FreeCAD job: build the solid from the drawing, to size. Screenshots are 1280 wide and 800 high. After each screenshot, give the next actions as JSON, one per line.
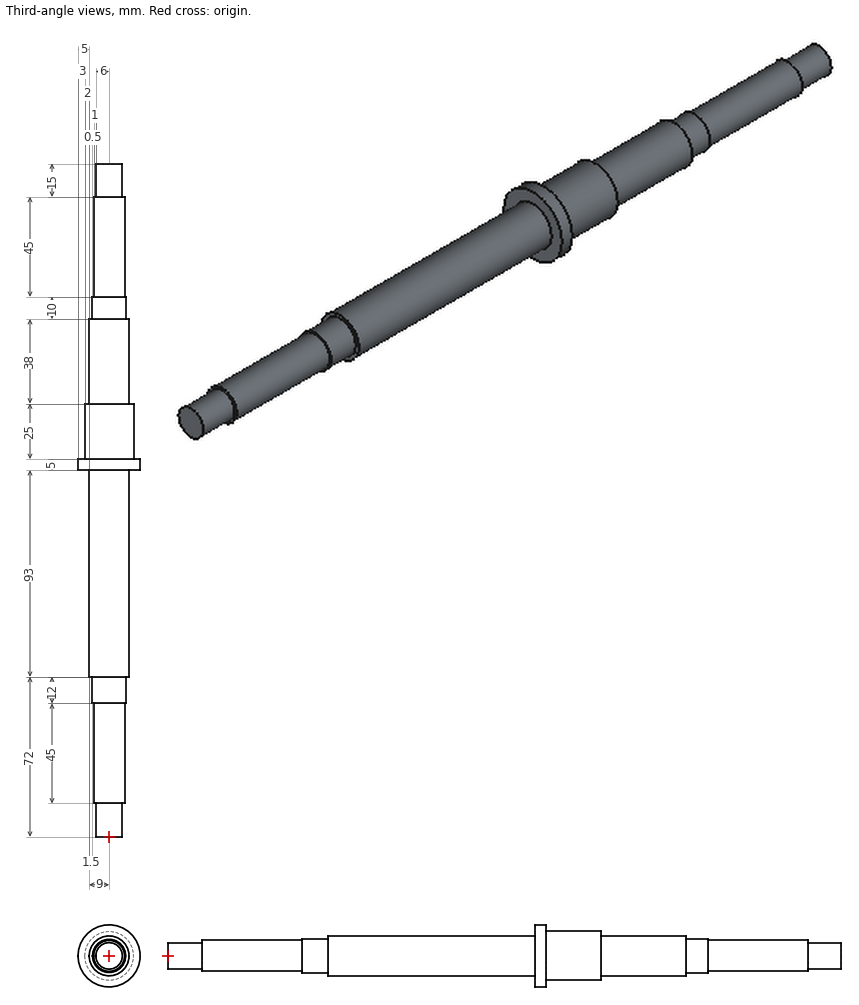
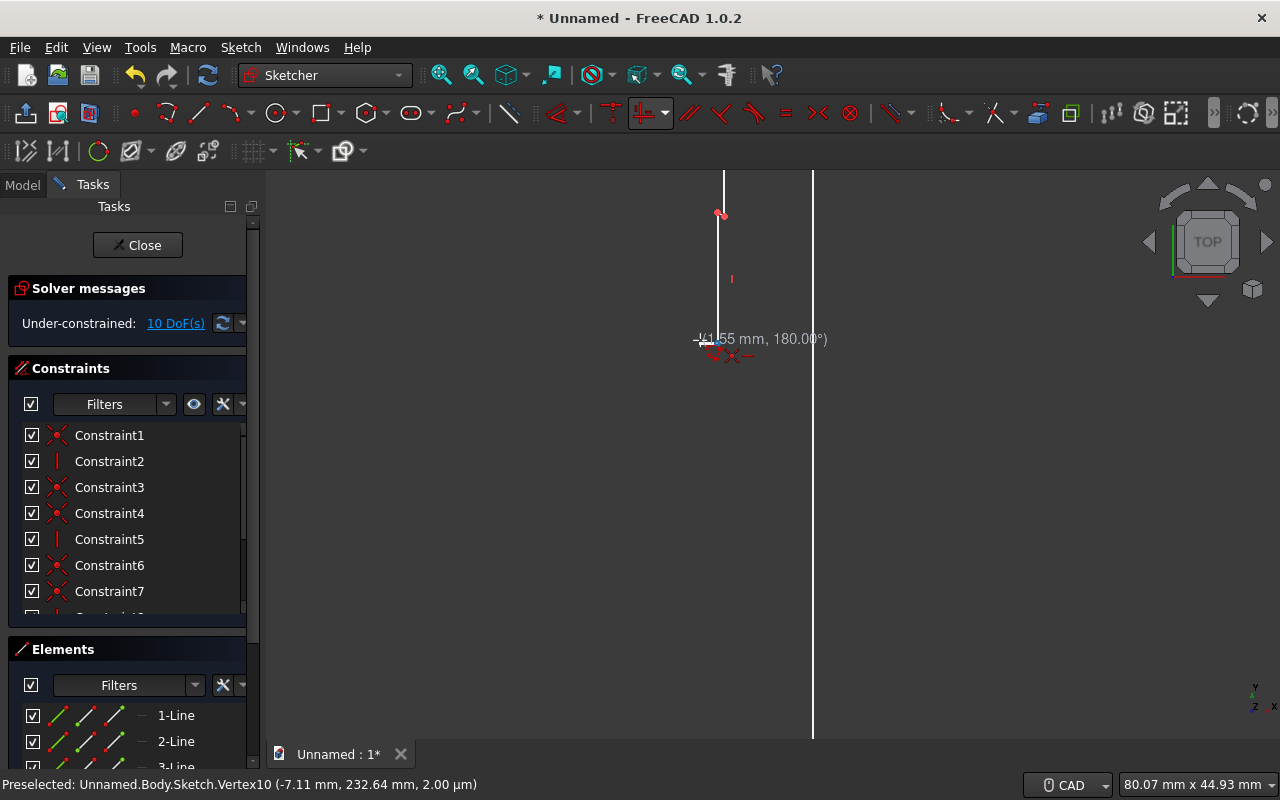
{"action": "left_click", "coordinate": [699, 339]}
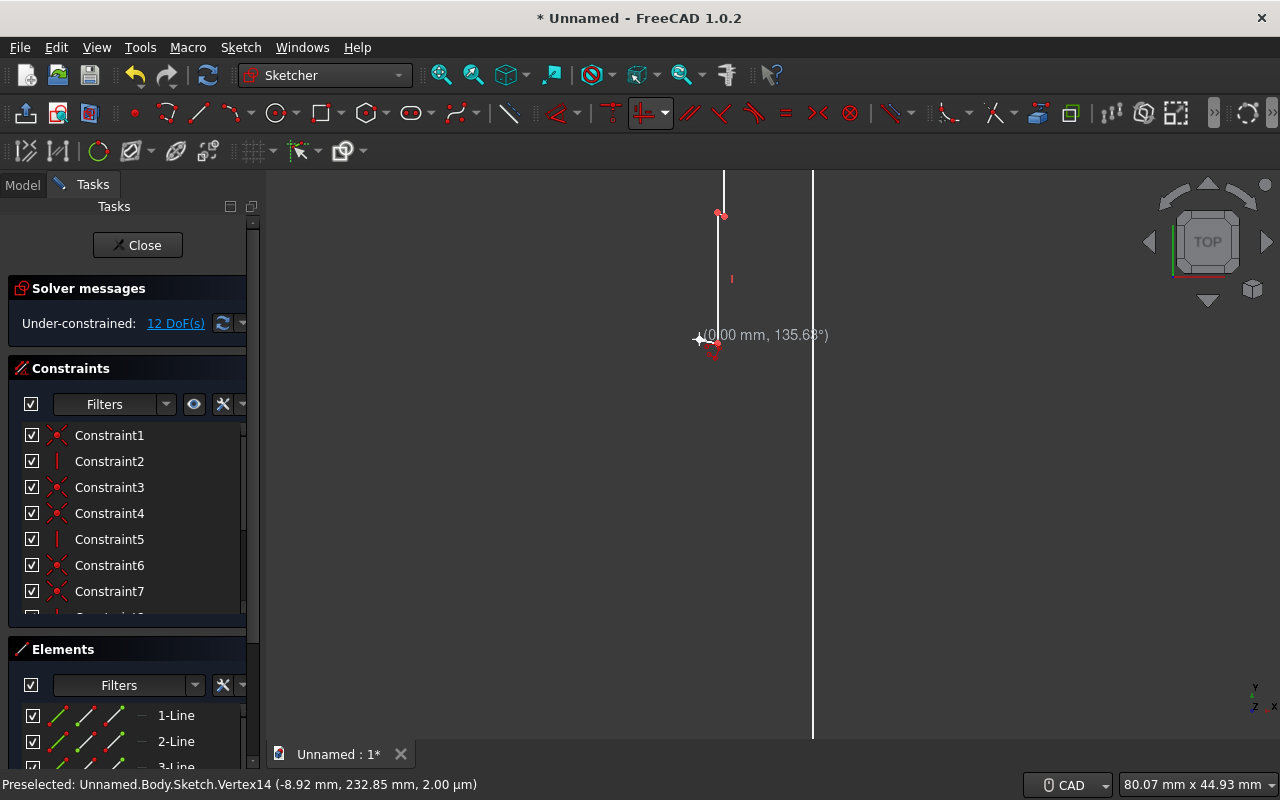
{"action": "scroll", "coordinate": [703, 363], "scroll_direction": "down", "scroll_amount": 12}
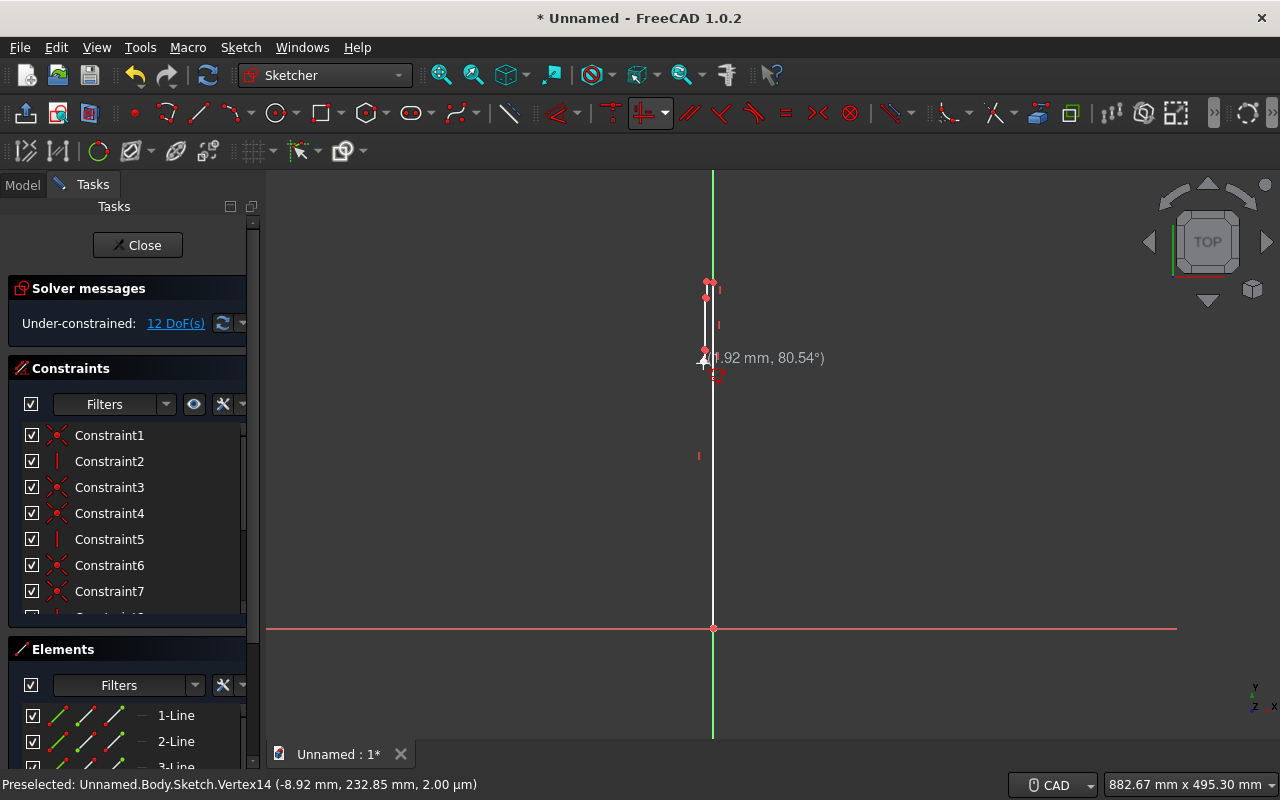
{"action": "scroll", "coordinate": [703, 405], "scroll_direction": "up", "scroll_amount": 3}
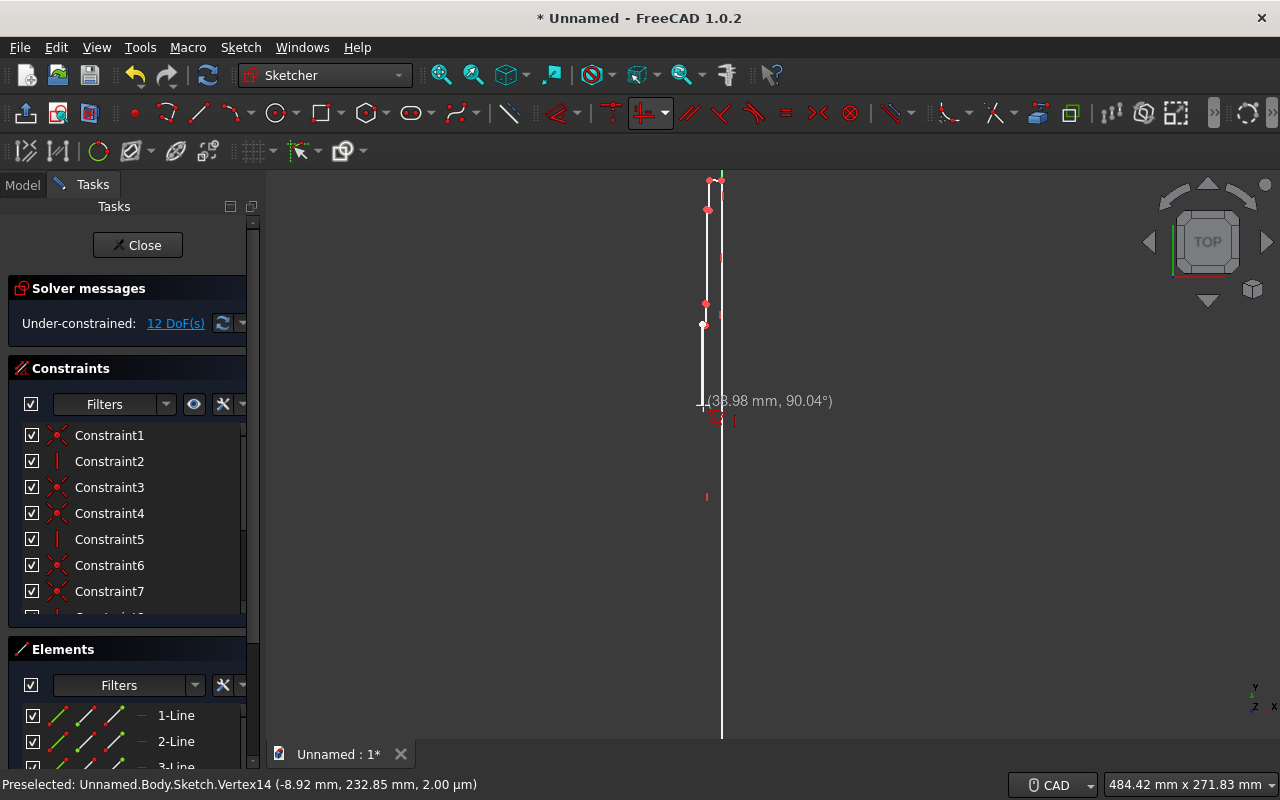
{"action": "left_click", "coordinate": [703, 404]}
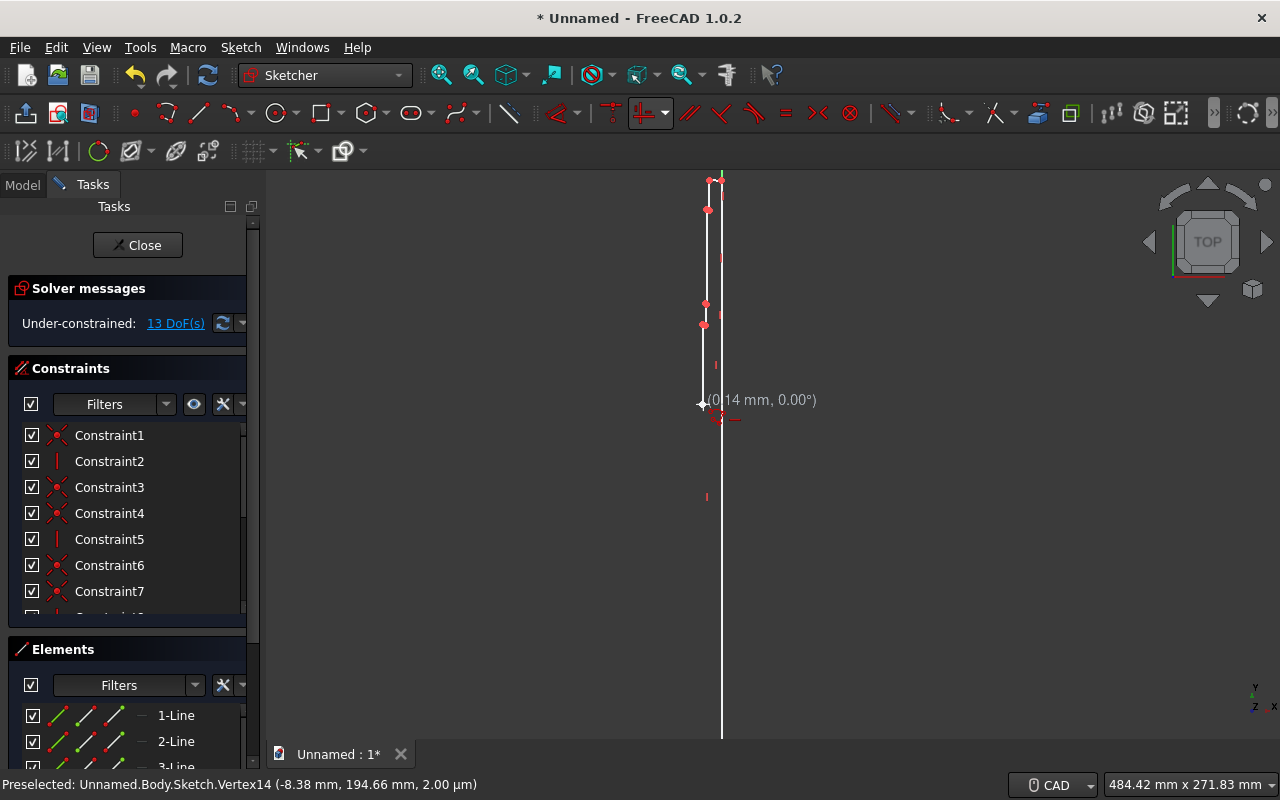
{"action": "scroll", "coordinate": [699, 404], "scroll_direction": "up", "scroll_amount": 7}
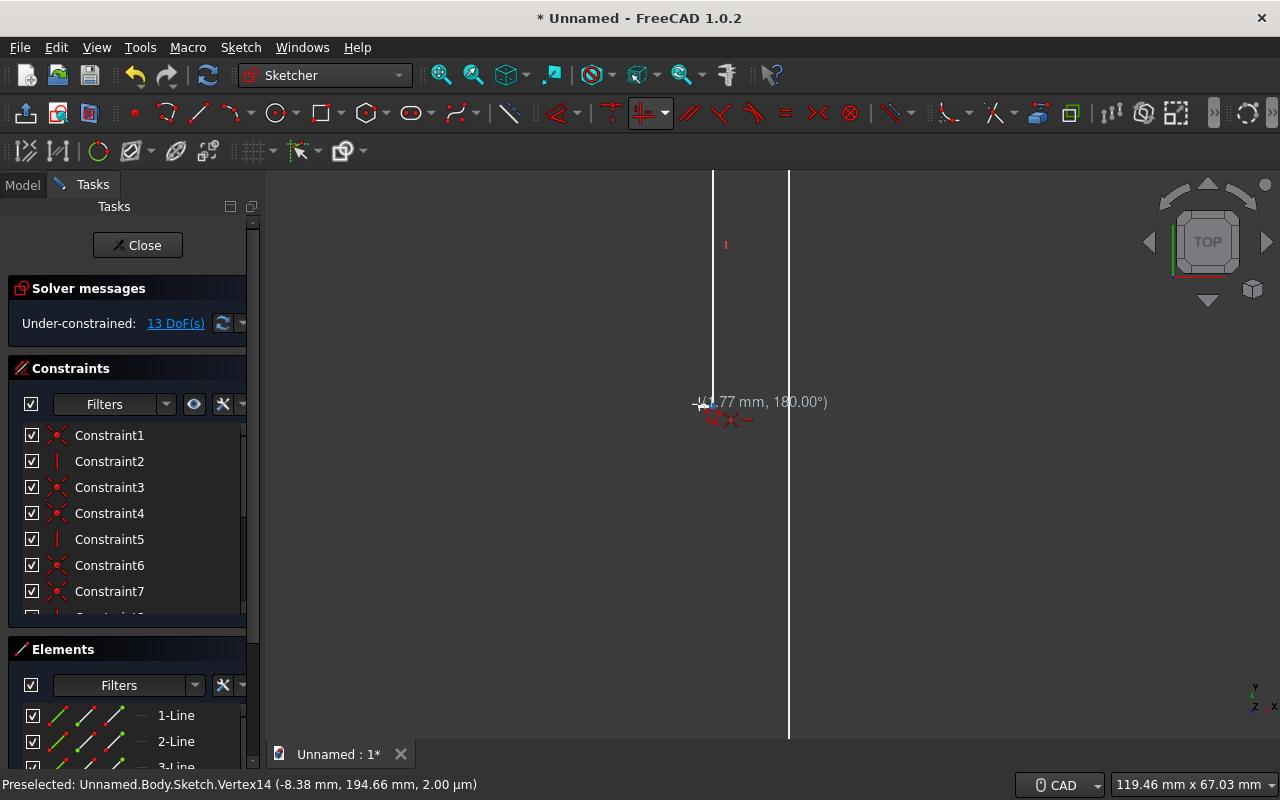
{"action": "left_click", "coordinate": [696, 403]}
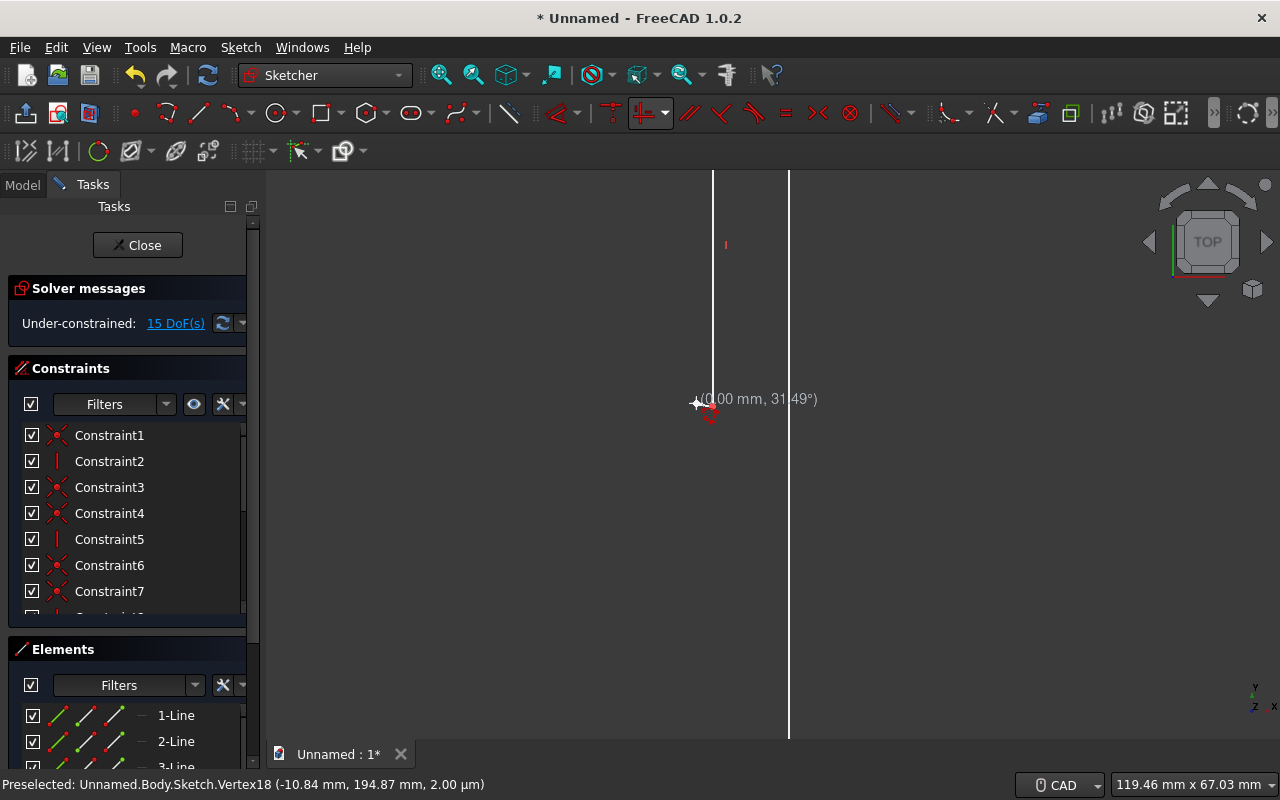
{"action": "scroll", "coordinate": [701, 405], "scroll_direction": "down", "scroll_amount": 10}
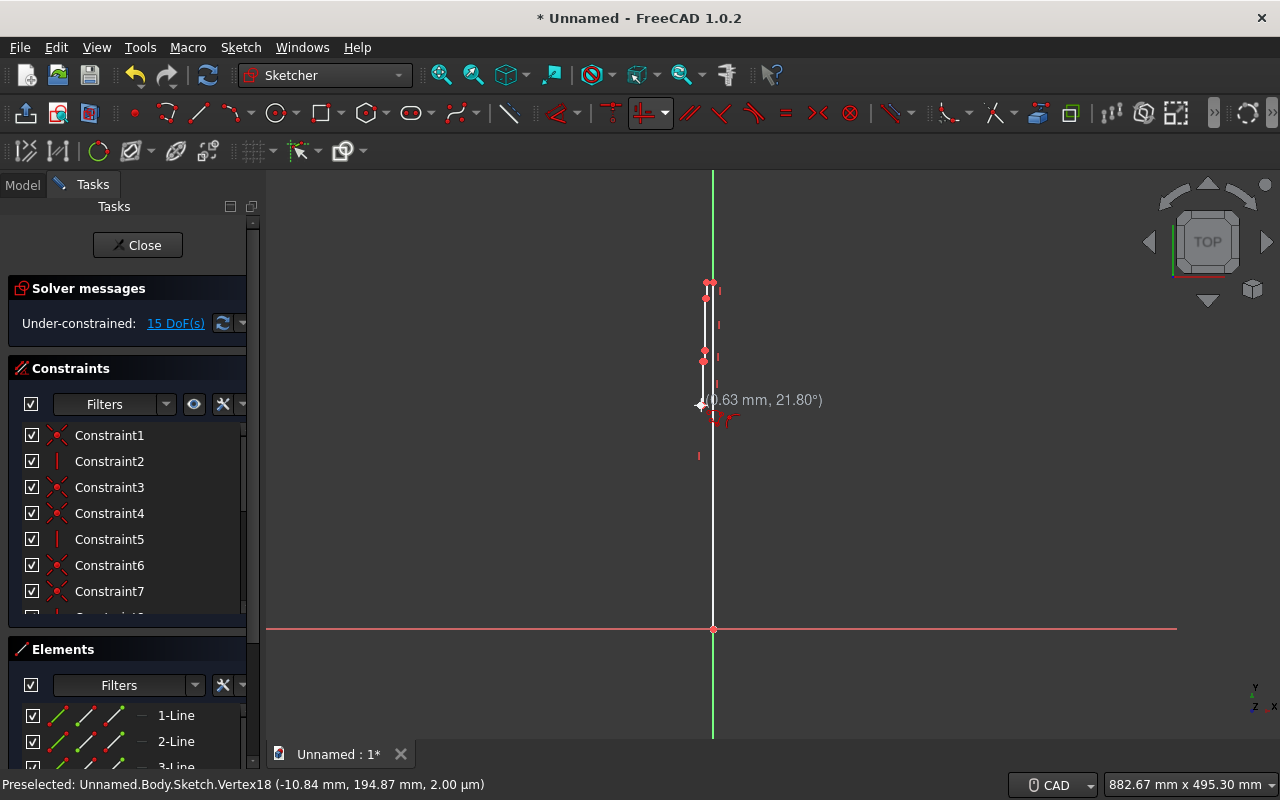
{"action": "scroll", "coordinate": [701, 434], "scroll_direction": "up", "scroll_amount": 2}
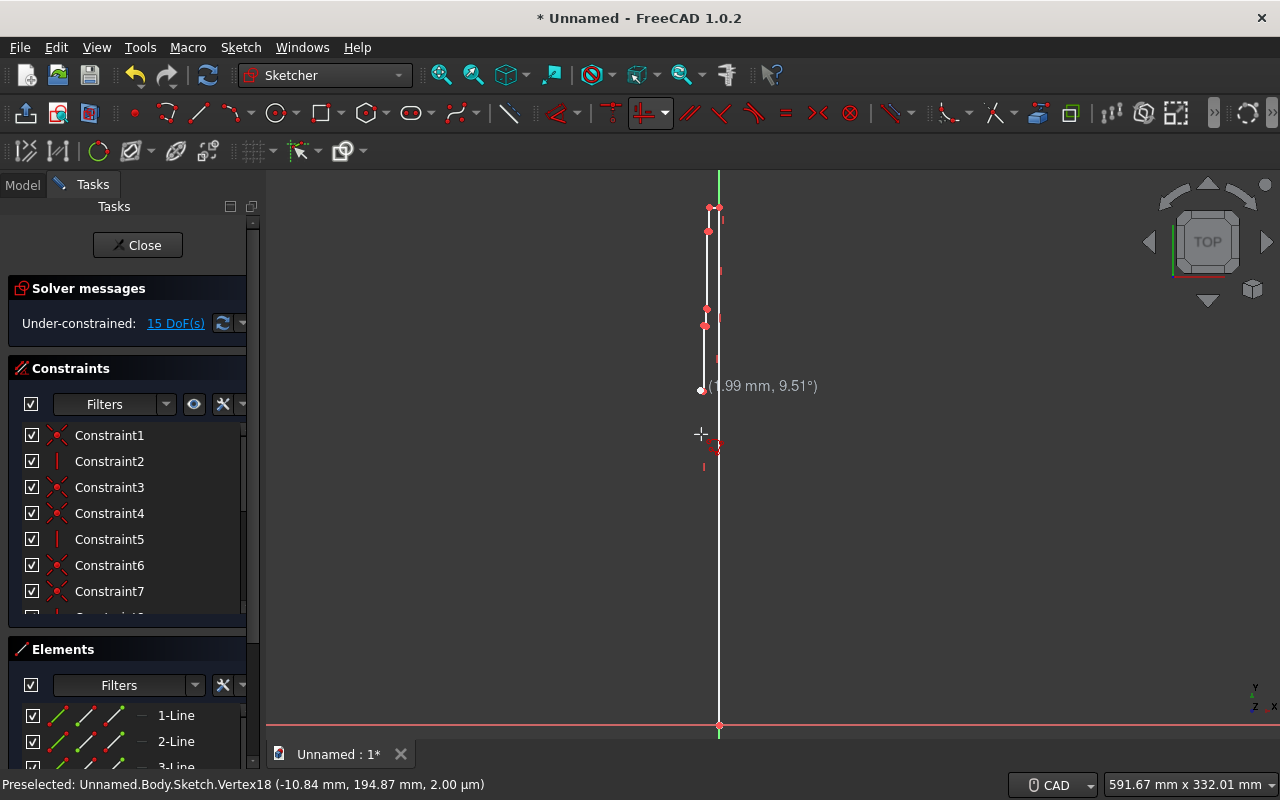
{"action": "left_click", "coordinate": [700, 434]}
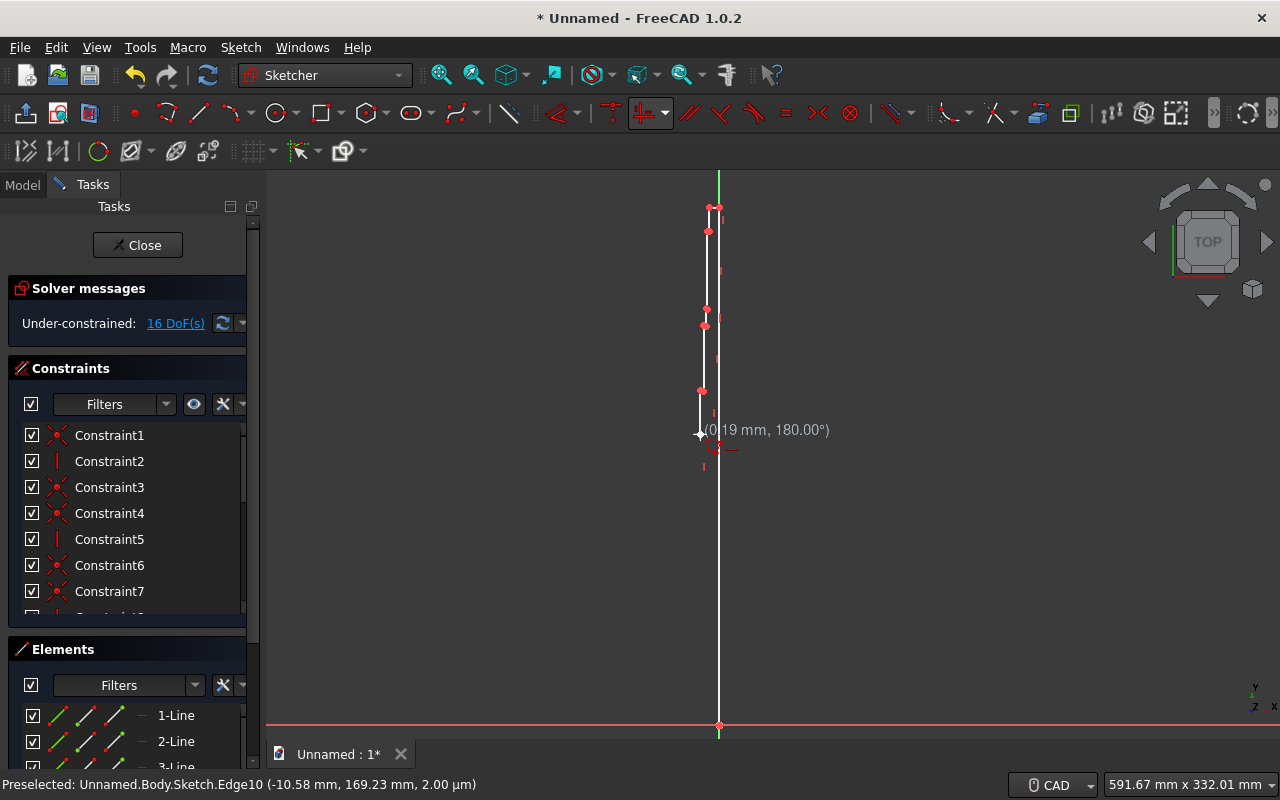
{"action": "scroll", "coordinate": [695, 434], "scroll_direction": "up", "scroll_amount": 6}